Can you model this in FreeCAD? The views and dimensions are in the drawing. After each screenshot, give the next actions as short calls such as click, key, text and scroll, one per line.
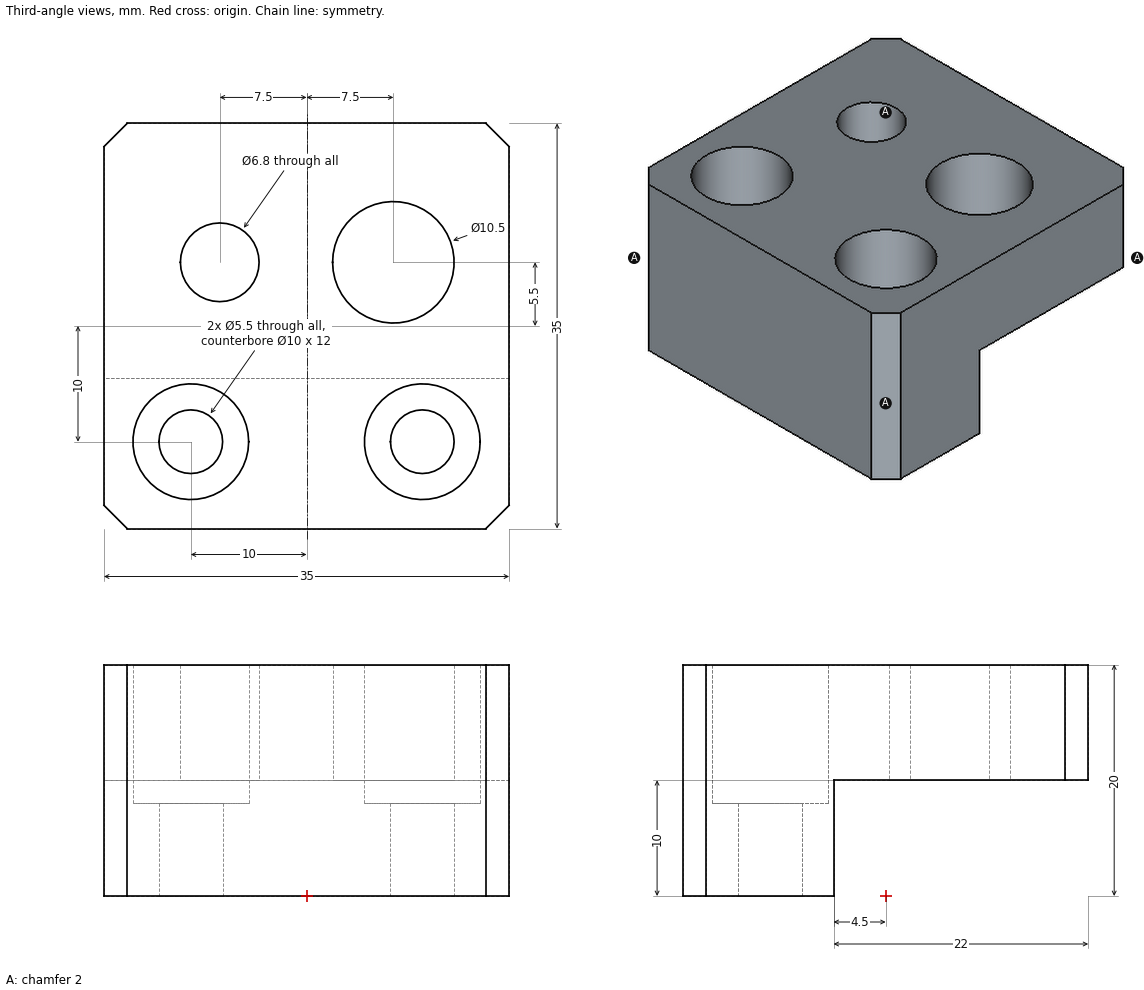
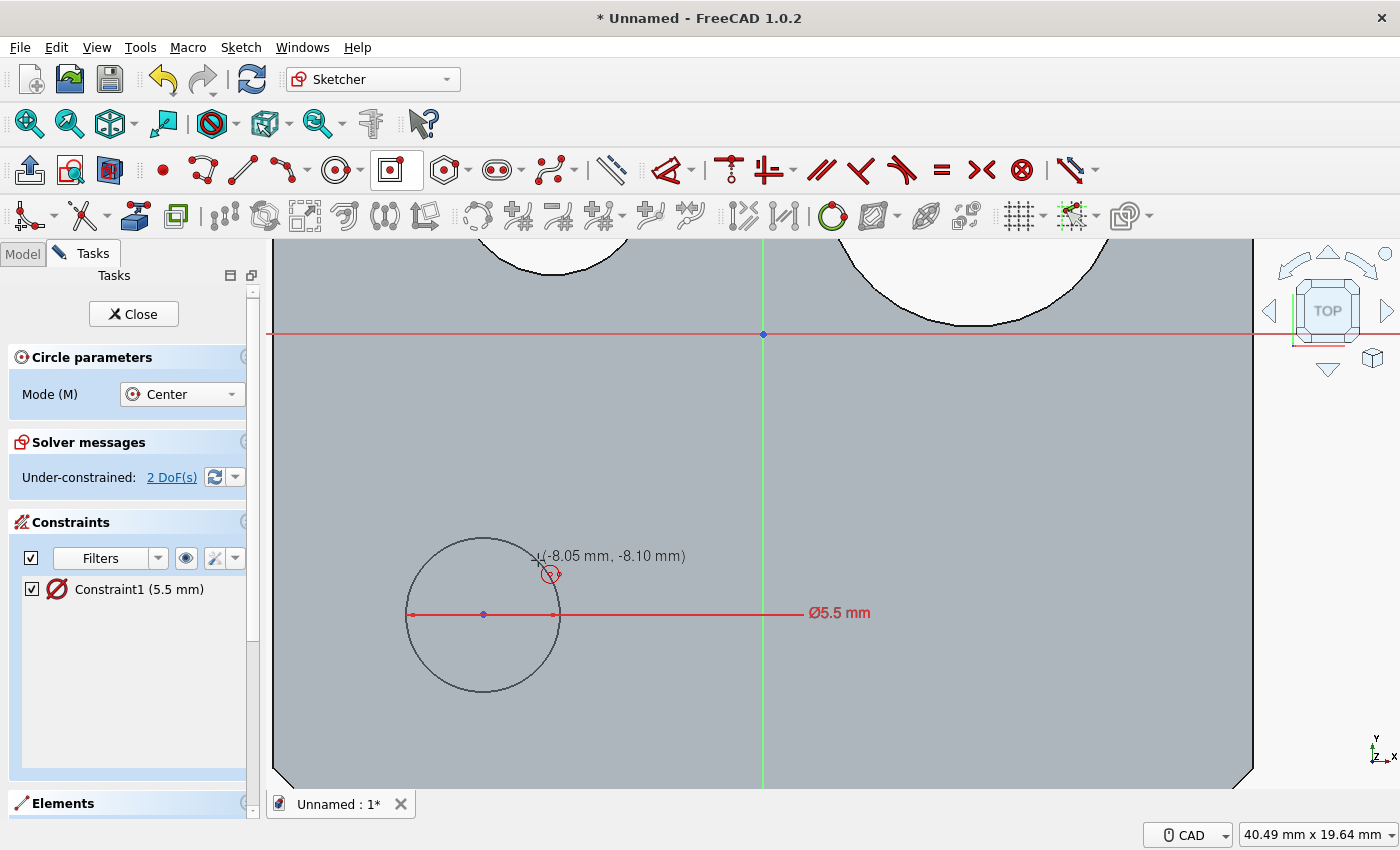
click(1043, 614)
move(1098, 560)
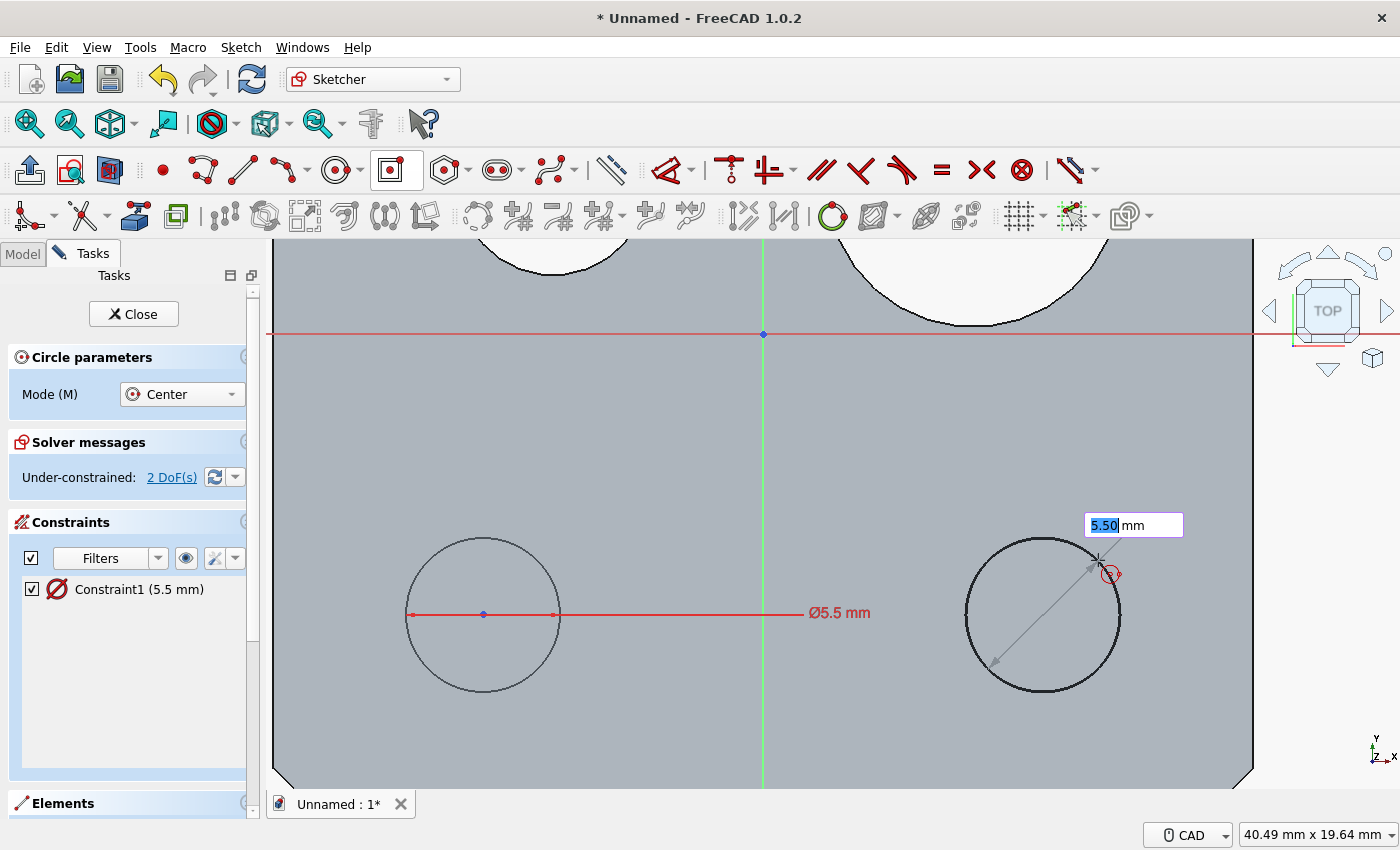
text(5.5)
key(Return)
key(Escape)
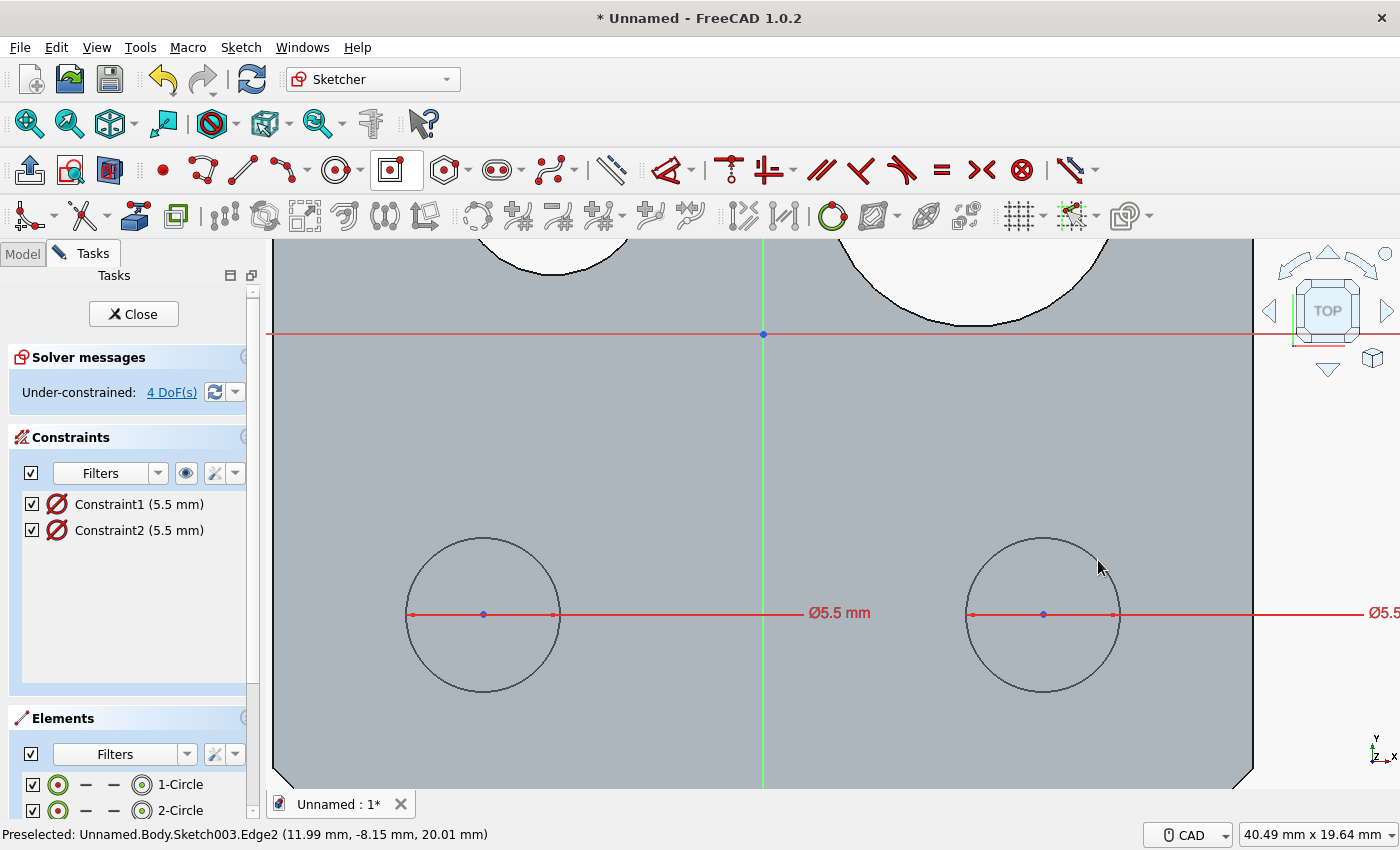
click(483, 615)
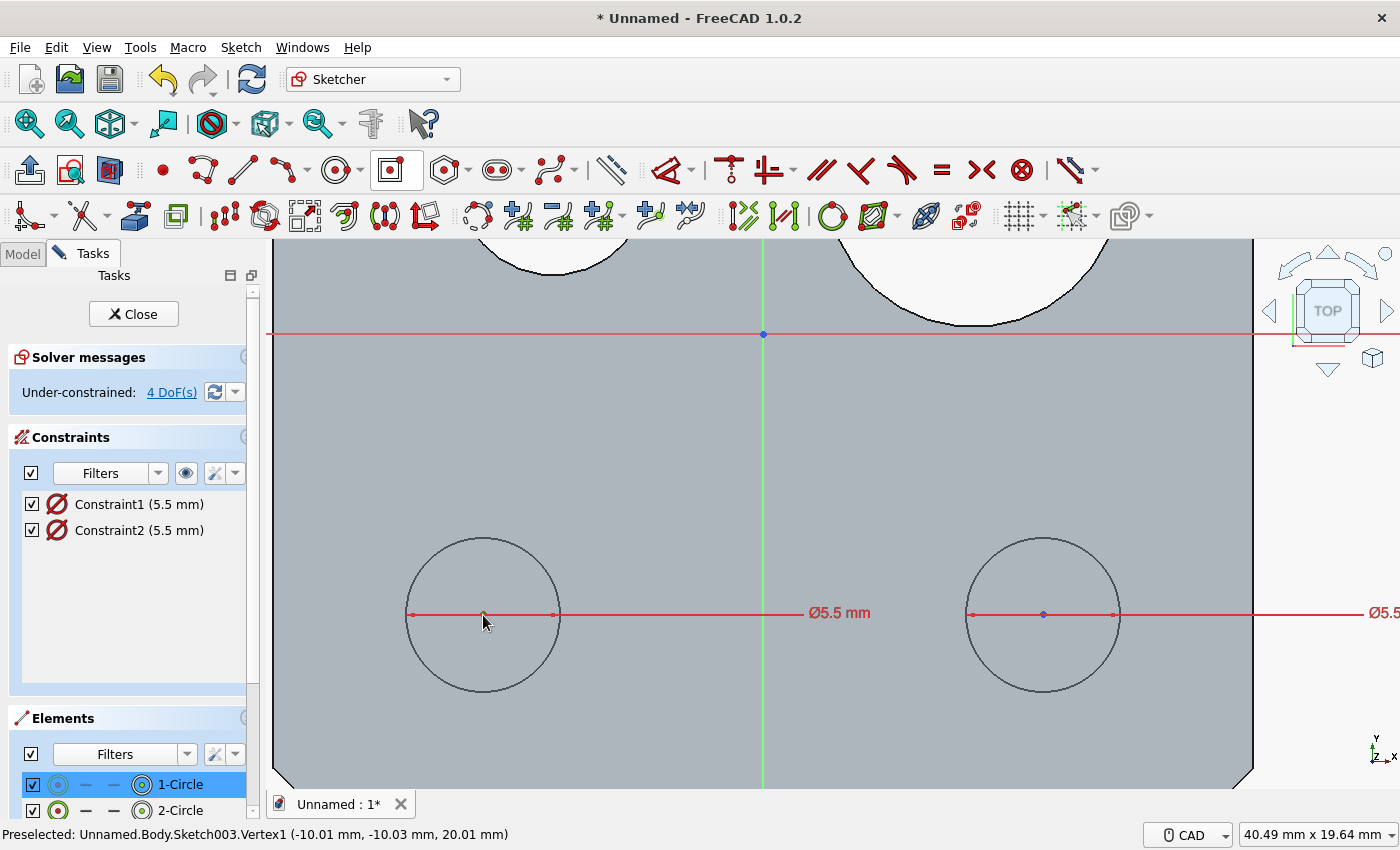
click(1043, 615)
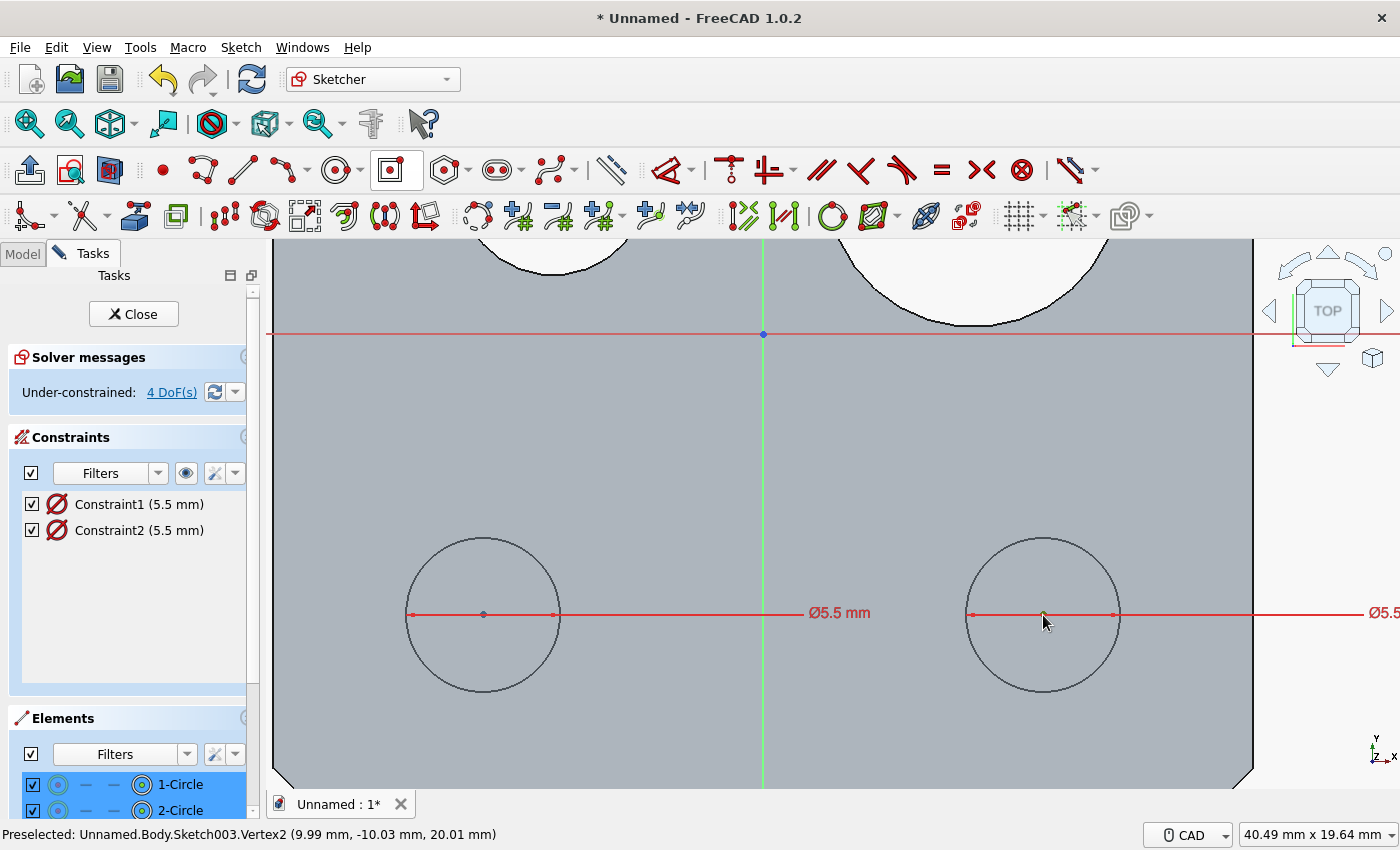
click(763, 726)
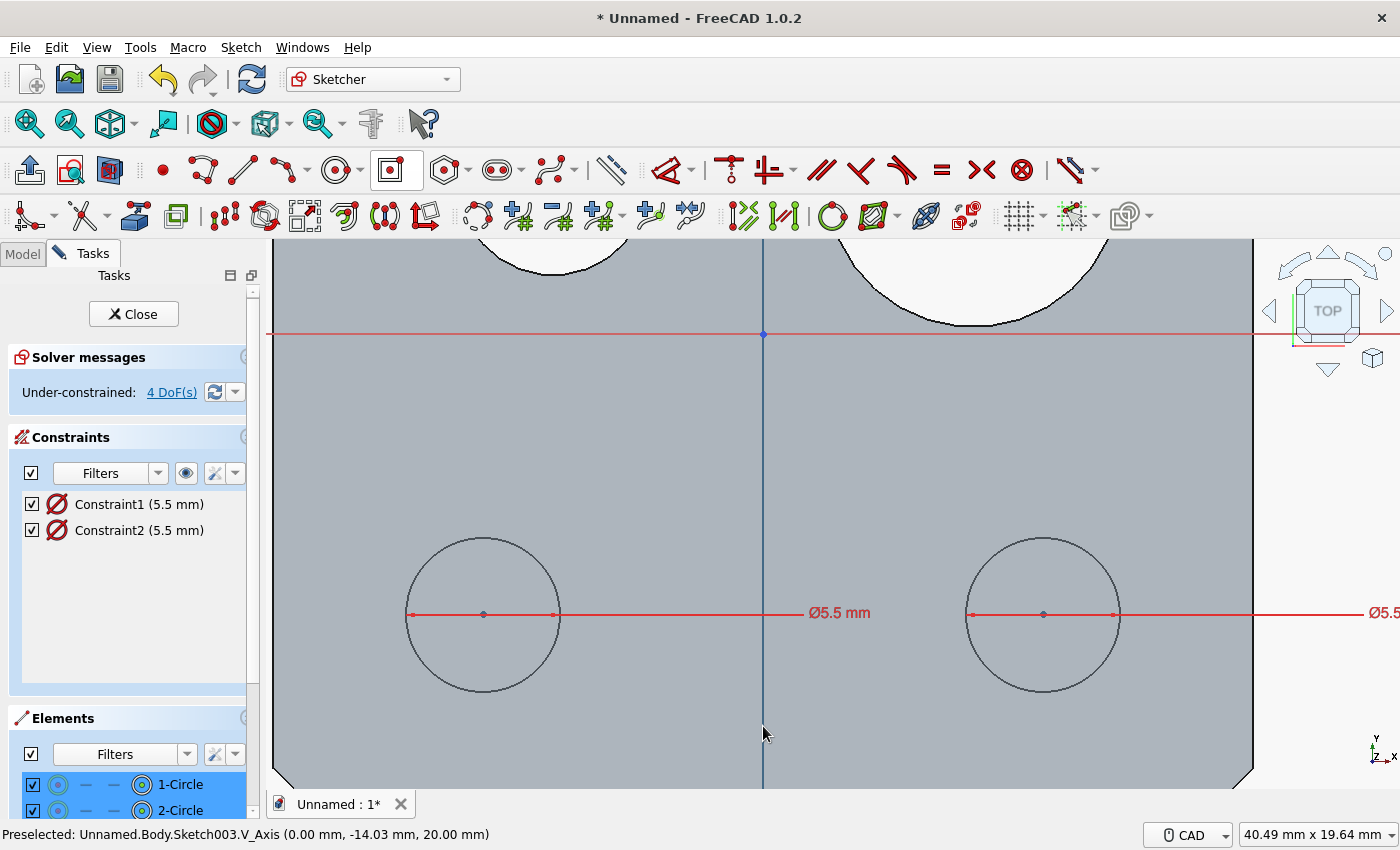
key(s)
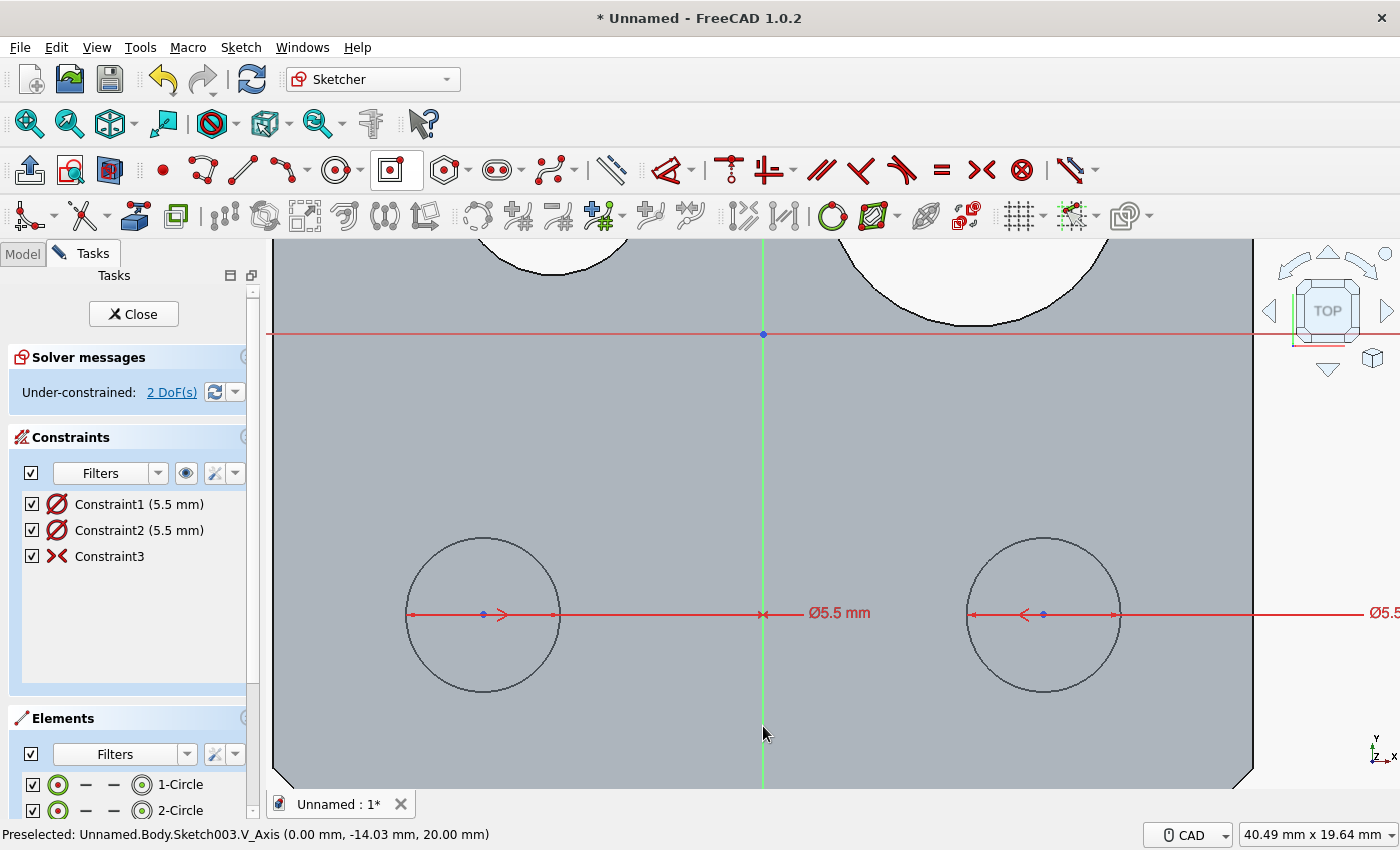
key(d)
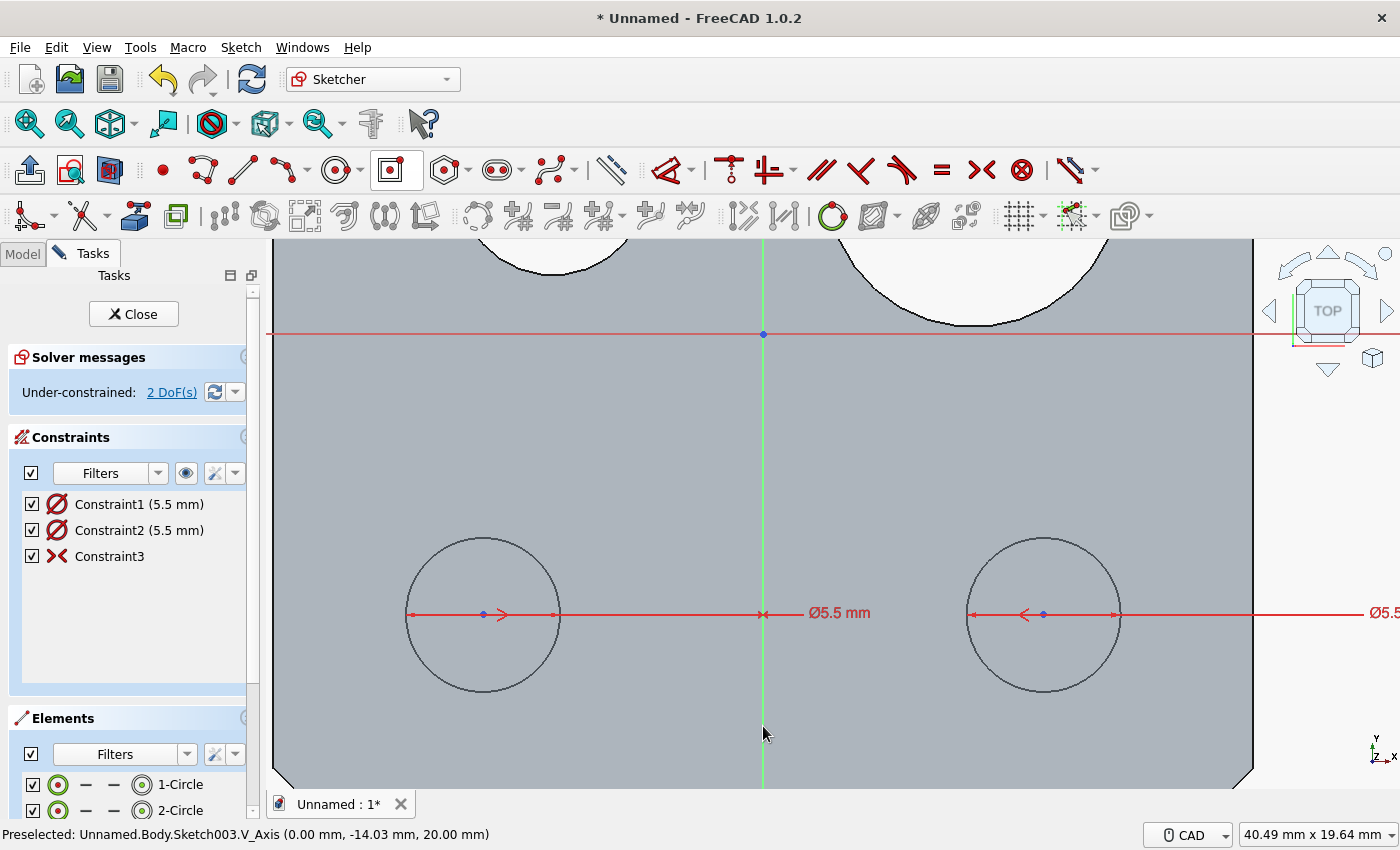
click(483, 615)
click(623, 300)